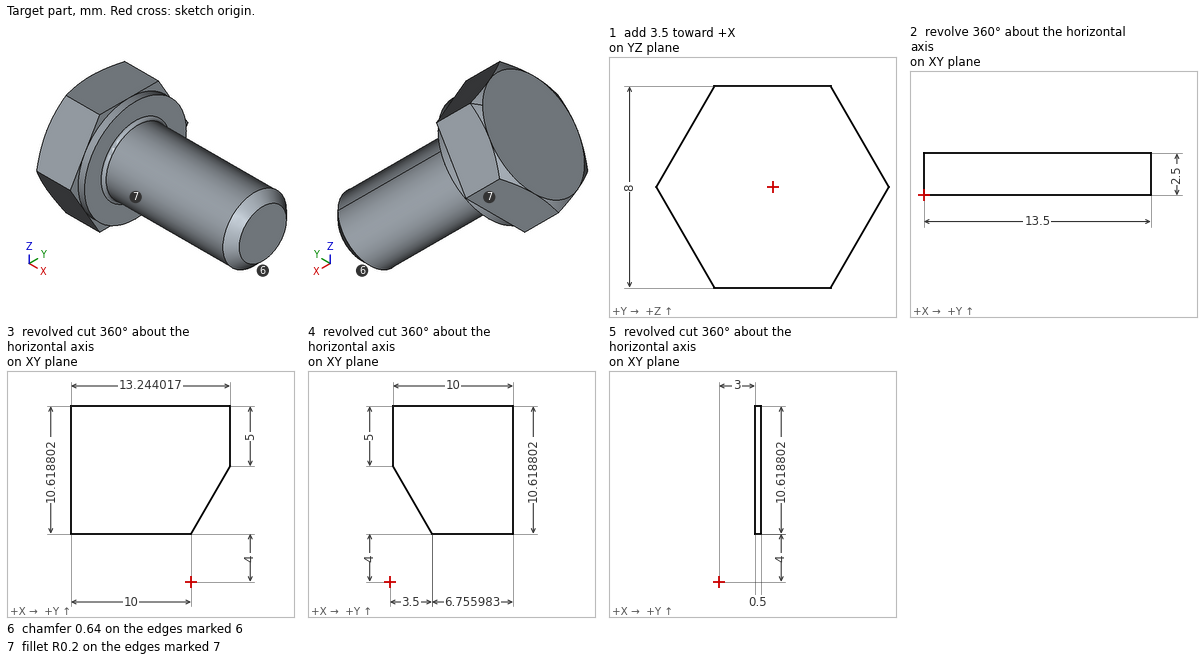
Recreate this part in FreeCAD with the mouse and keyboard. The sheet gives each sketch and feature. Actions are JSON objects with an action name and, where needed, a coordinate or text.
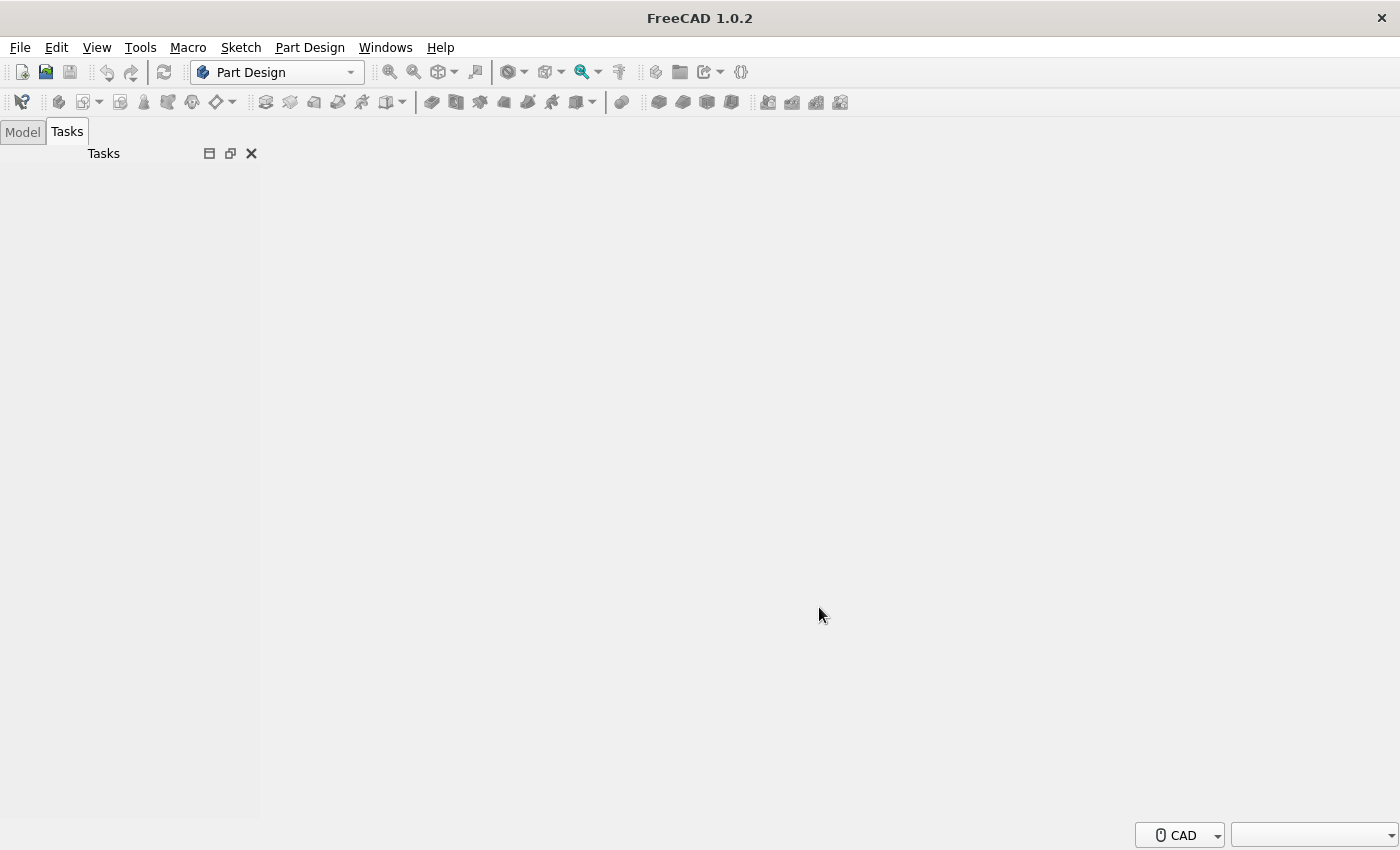
{"action": "left_click", "coordinate": [22, 72]}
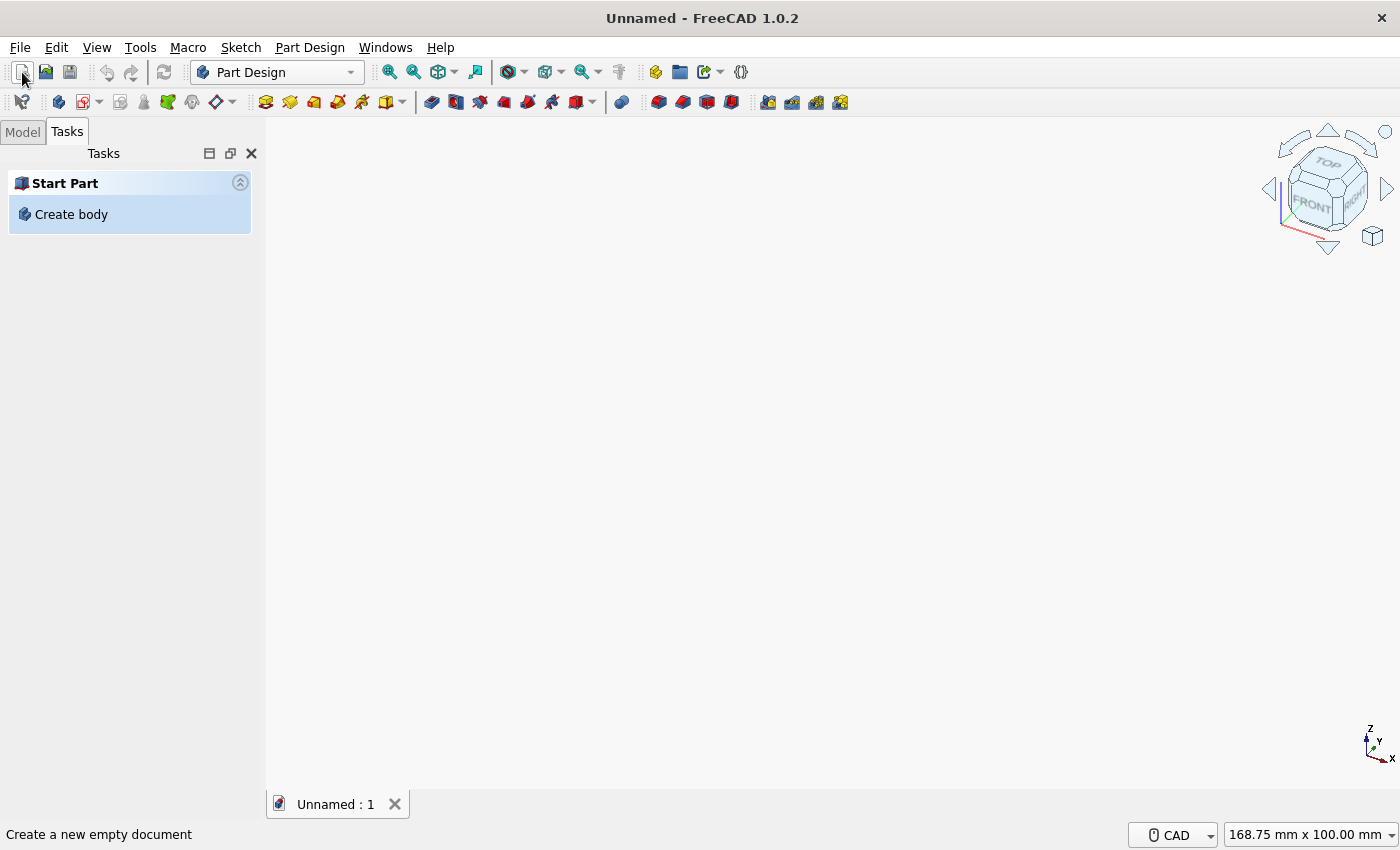
{"action": "left_click", "coordinate": [84, 102]}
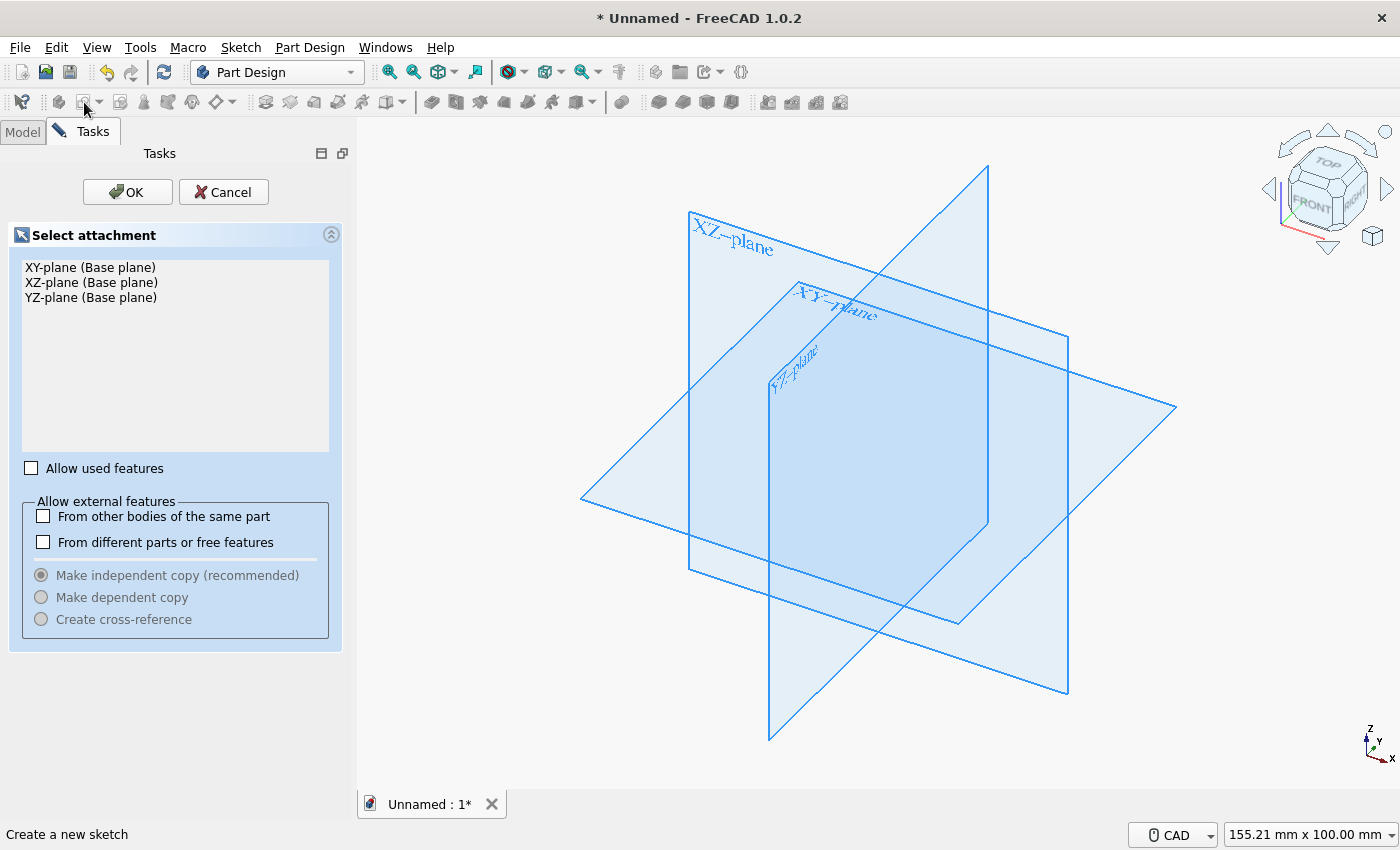
{"action": "left_click", "coordinate": [82, 298]}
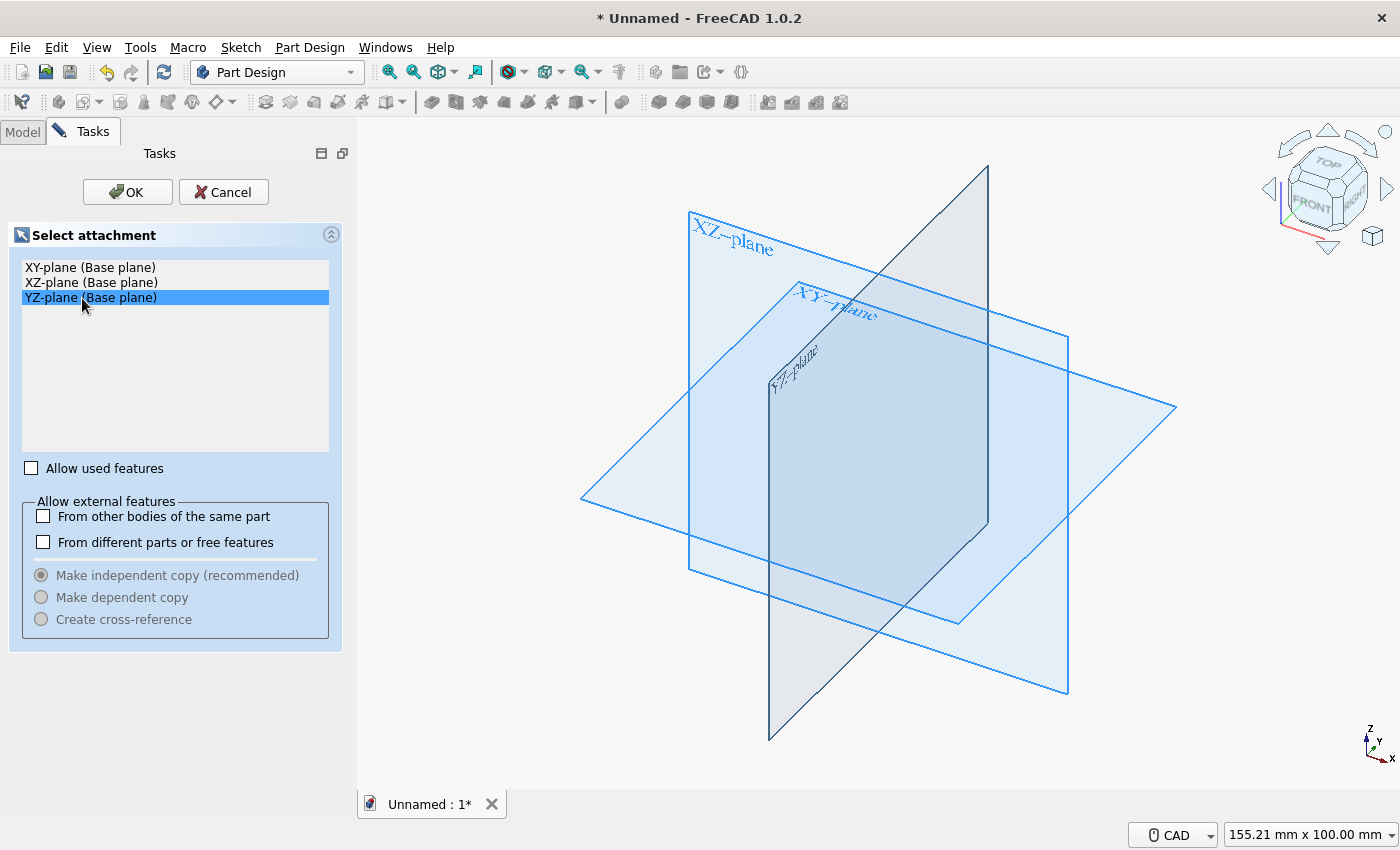
{"action": "left_click", "coordinate": [128, 192]}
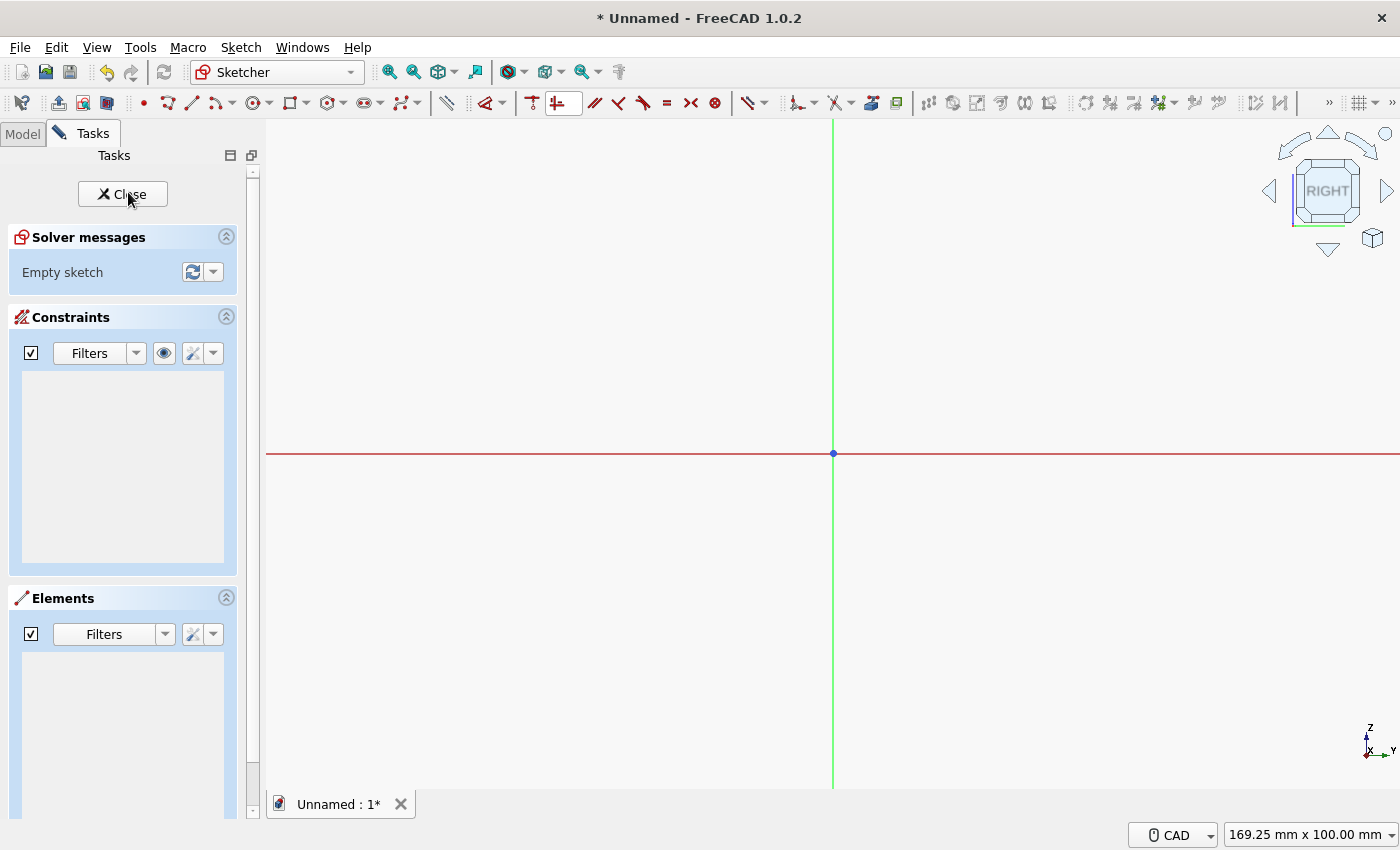
{"action": "scroll", "coordinate": [844, 454], "scroll_direction": "up", "scroll_amount": 10}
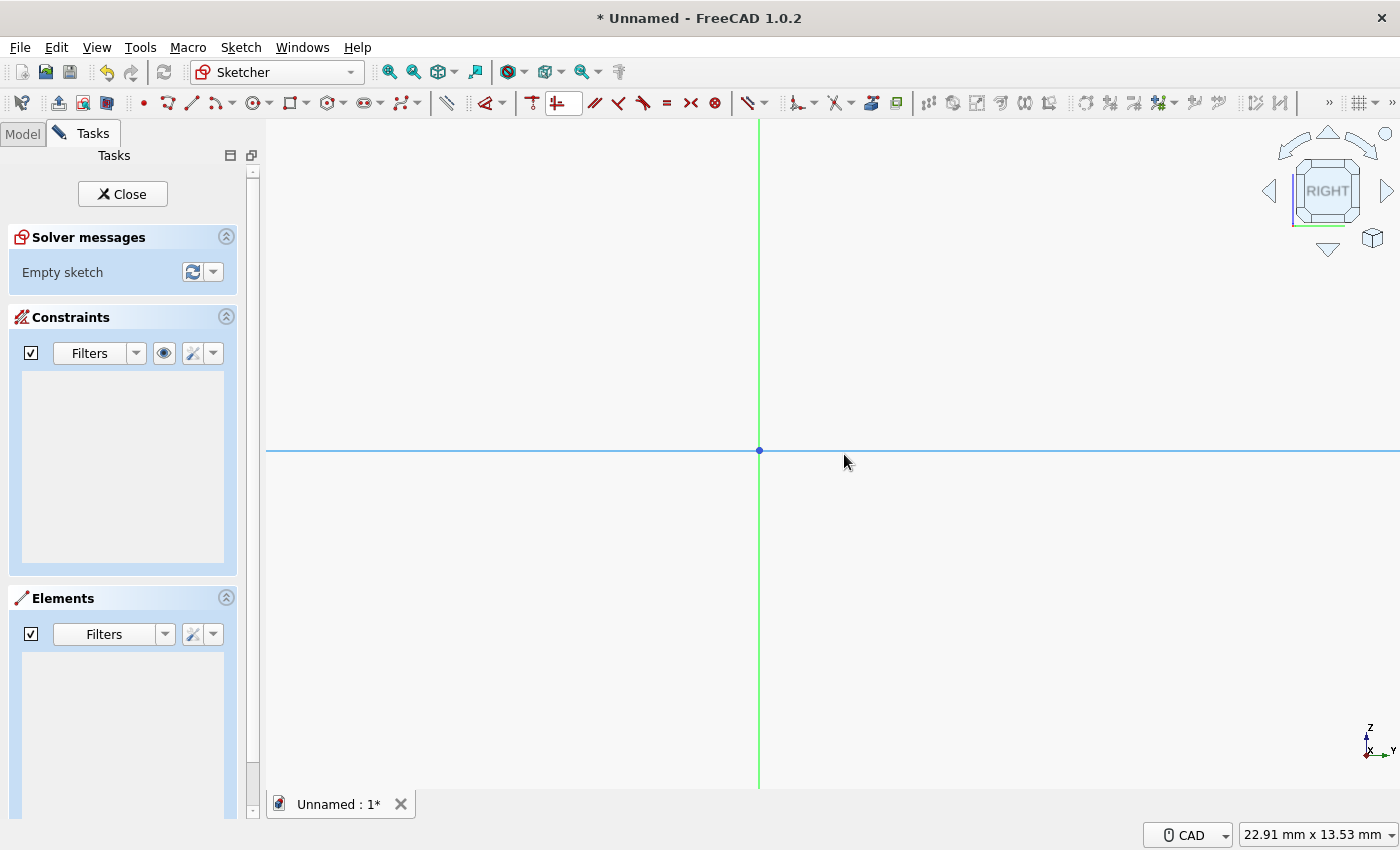
{"action": "left_click", "coordinate": [328, 104]}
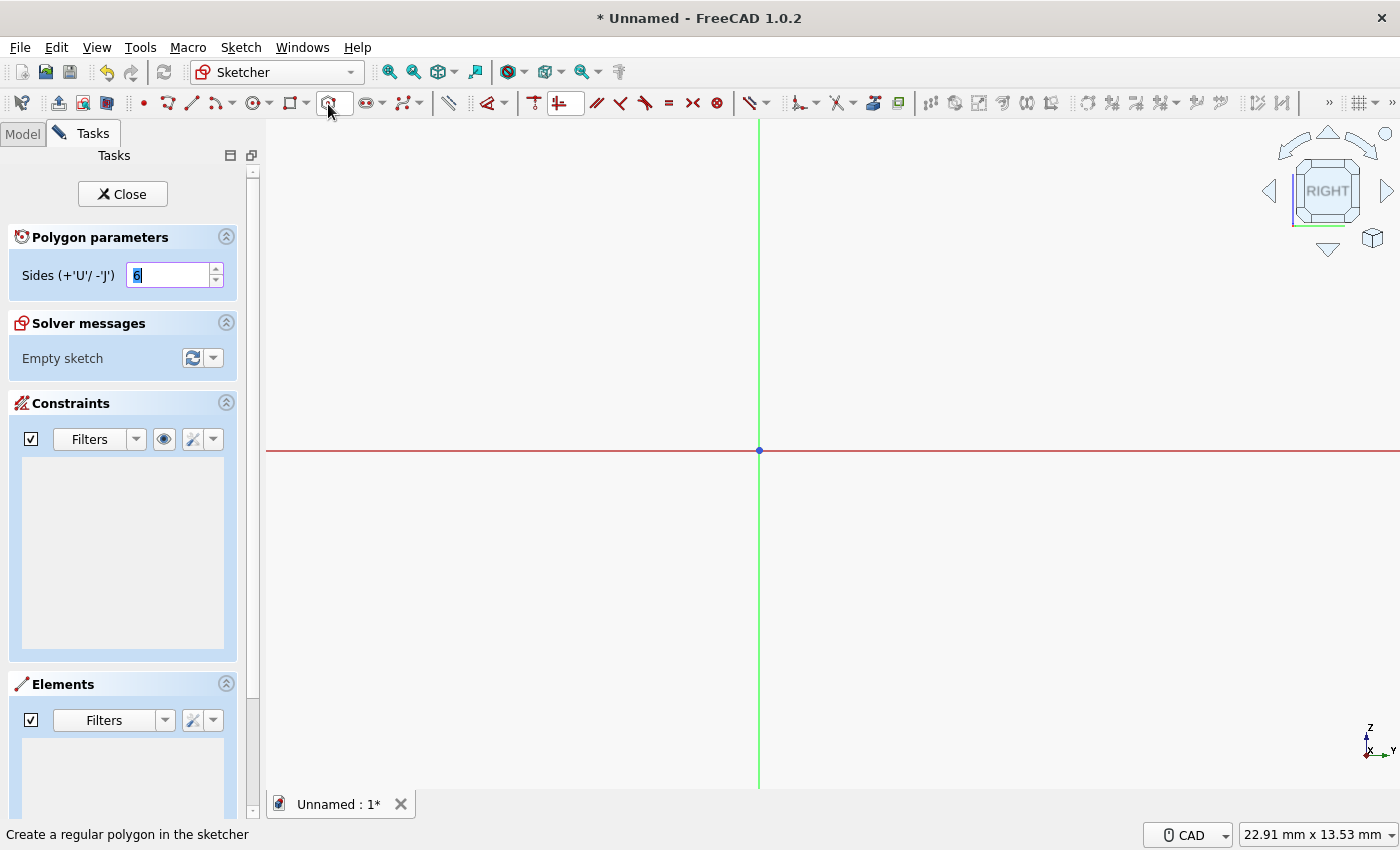
{"action": "left_click", "coordinate": [759, 451]}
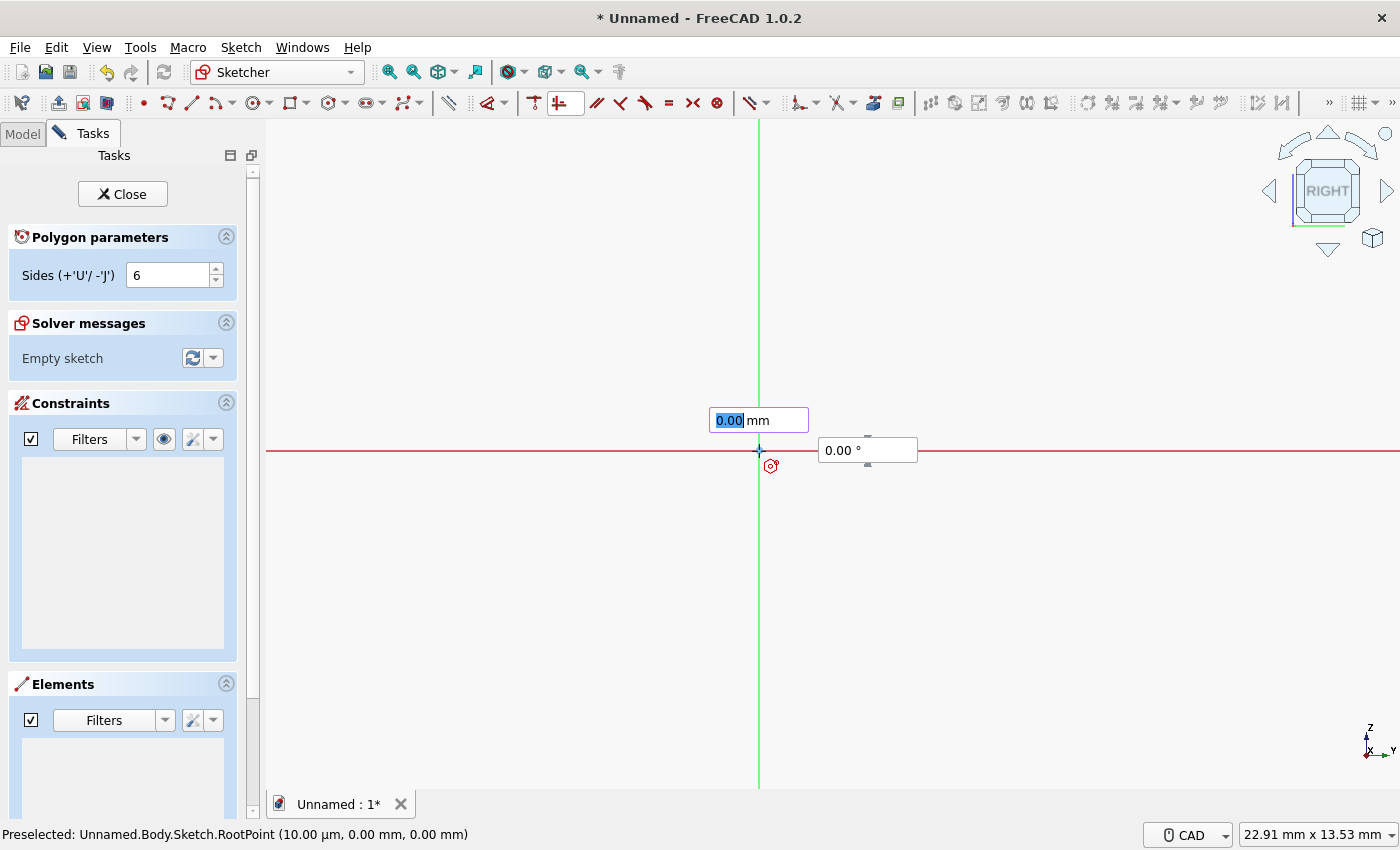
{"action": "left_click", "coordinate": [988, 451]}
{"action": "key", "text": "Escape"}